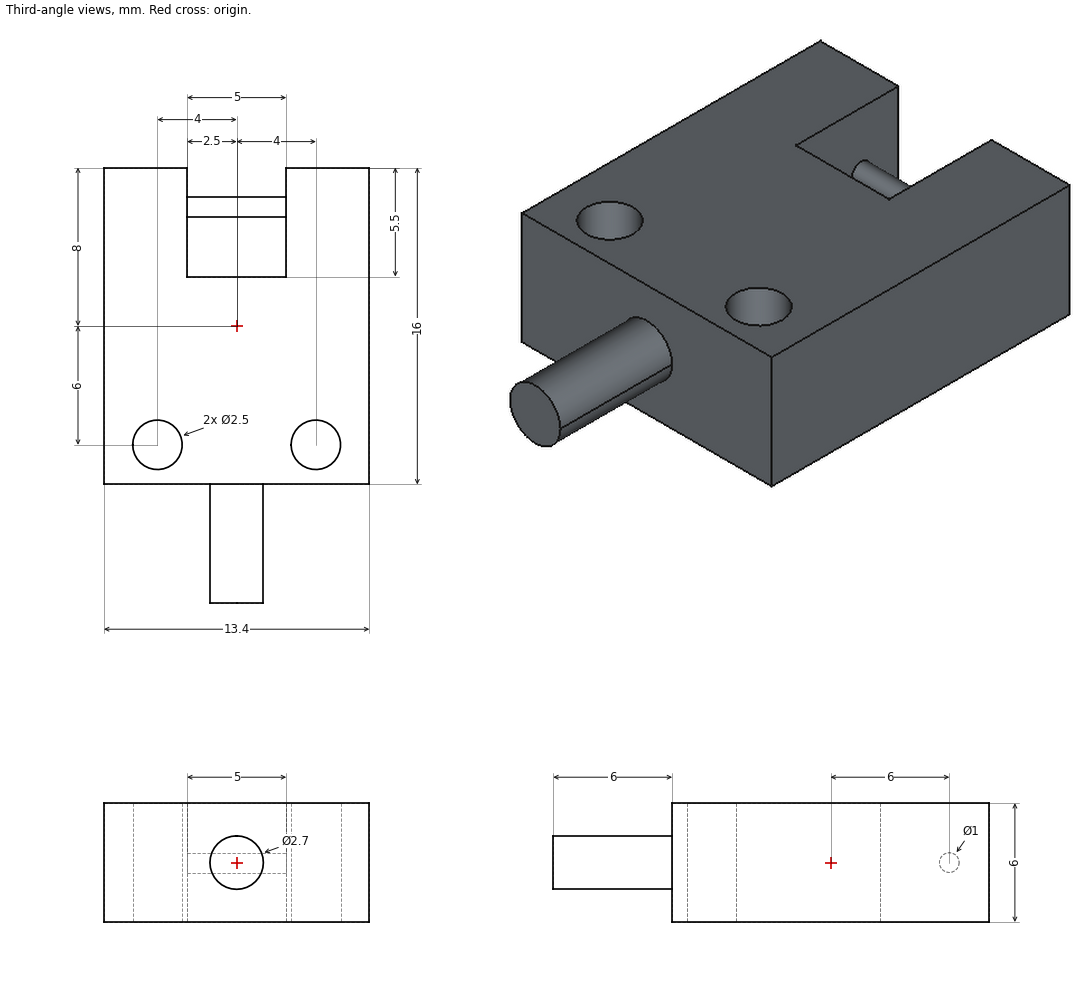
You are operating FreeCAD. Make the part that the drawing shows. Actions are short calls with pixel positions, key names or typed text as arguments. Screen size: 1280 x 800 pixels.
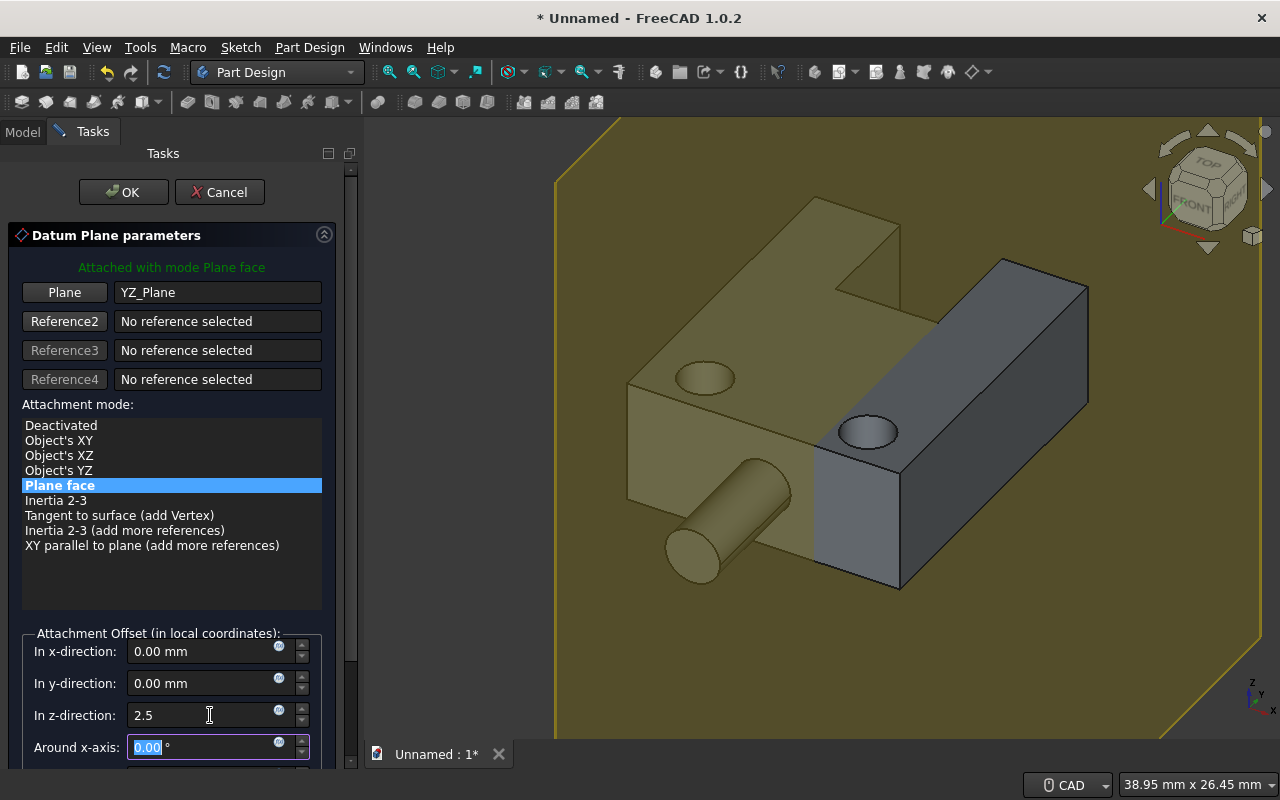
click(124, 192)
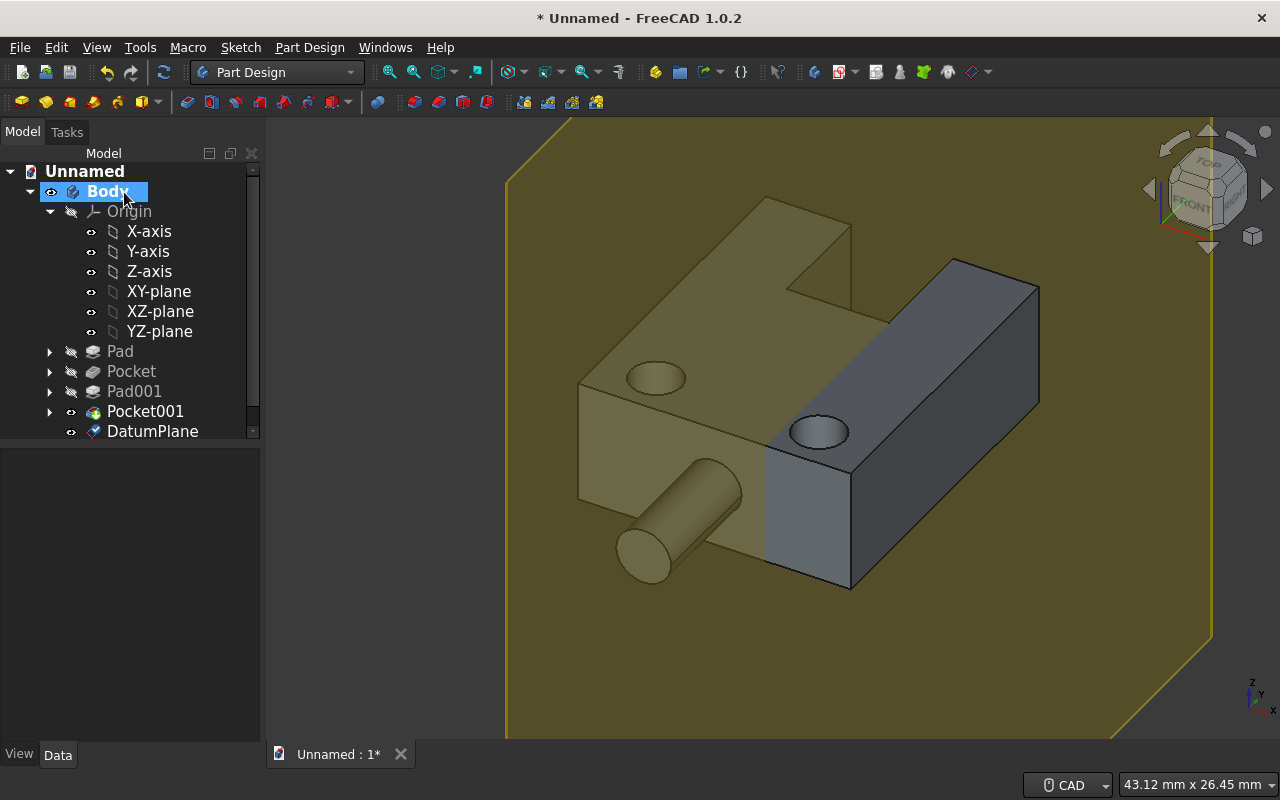
click(116, 432)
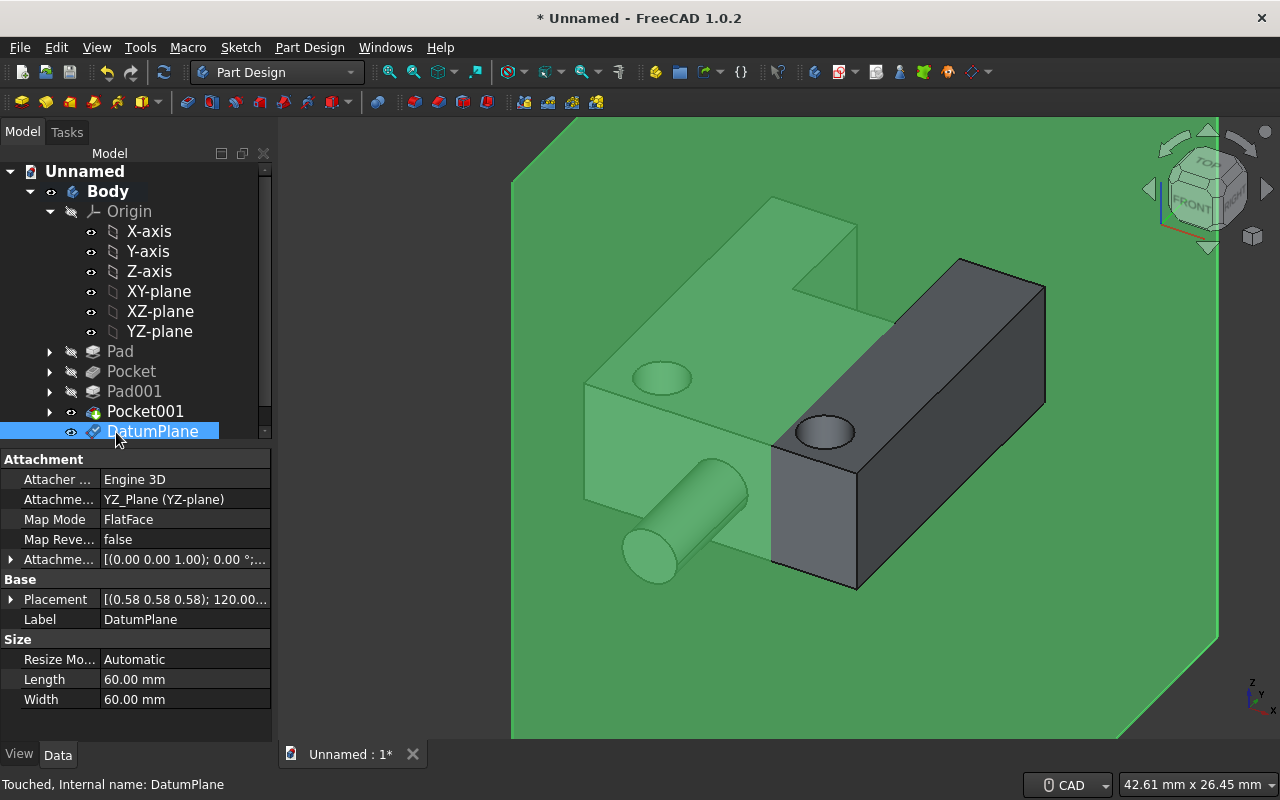
click(840, 72)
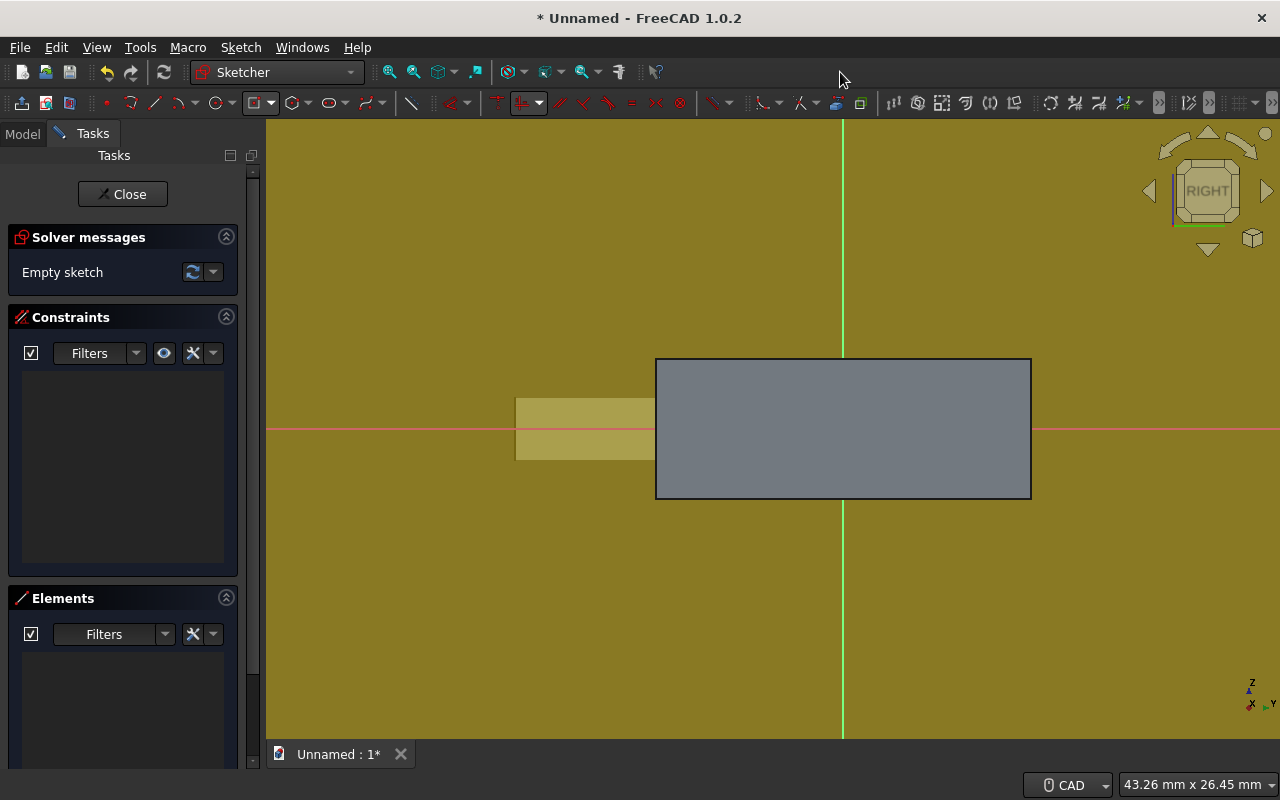
key(q)
key(s)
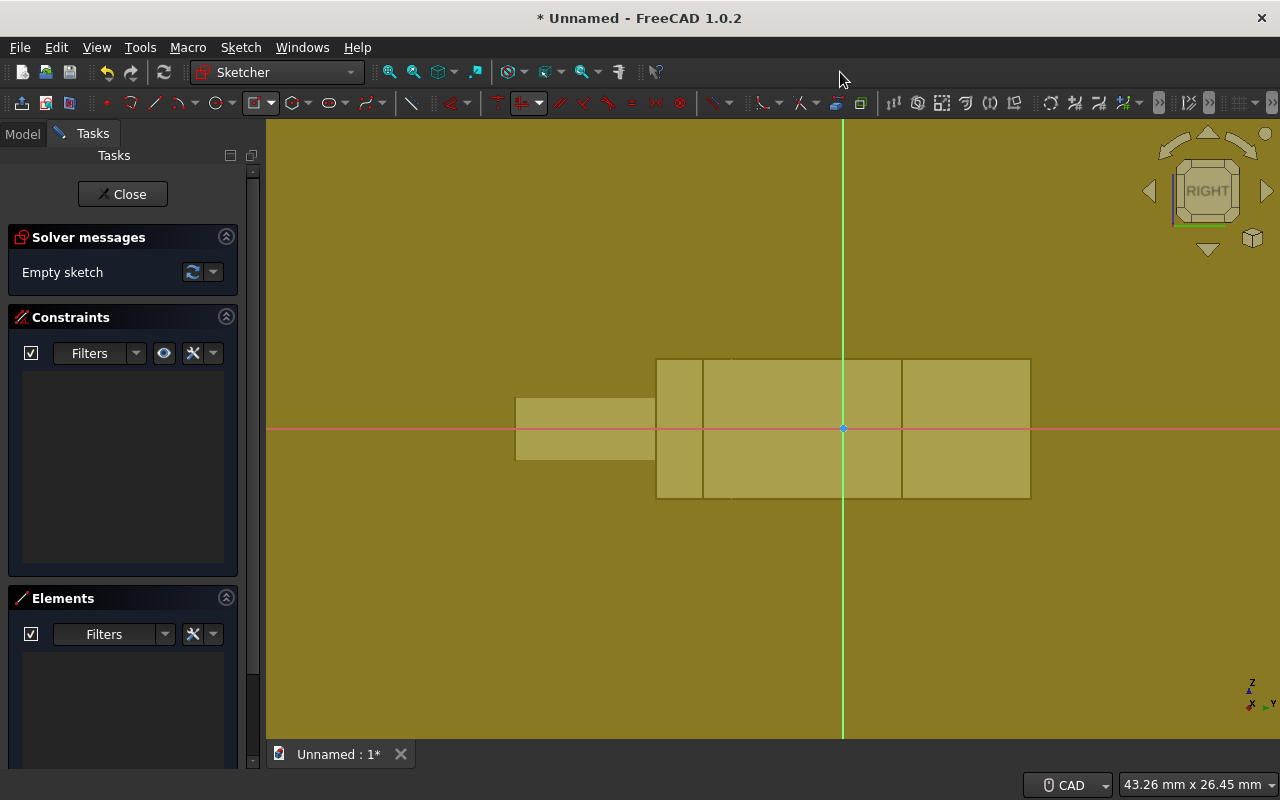
scroll(1002, 429, up, 14)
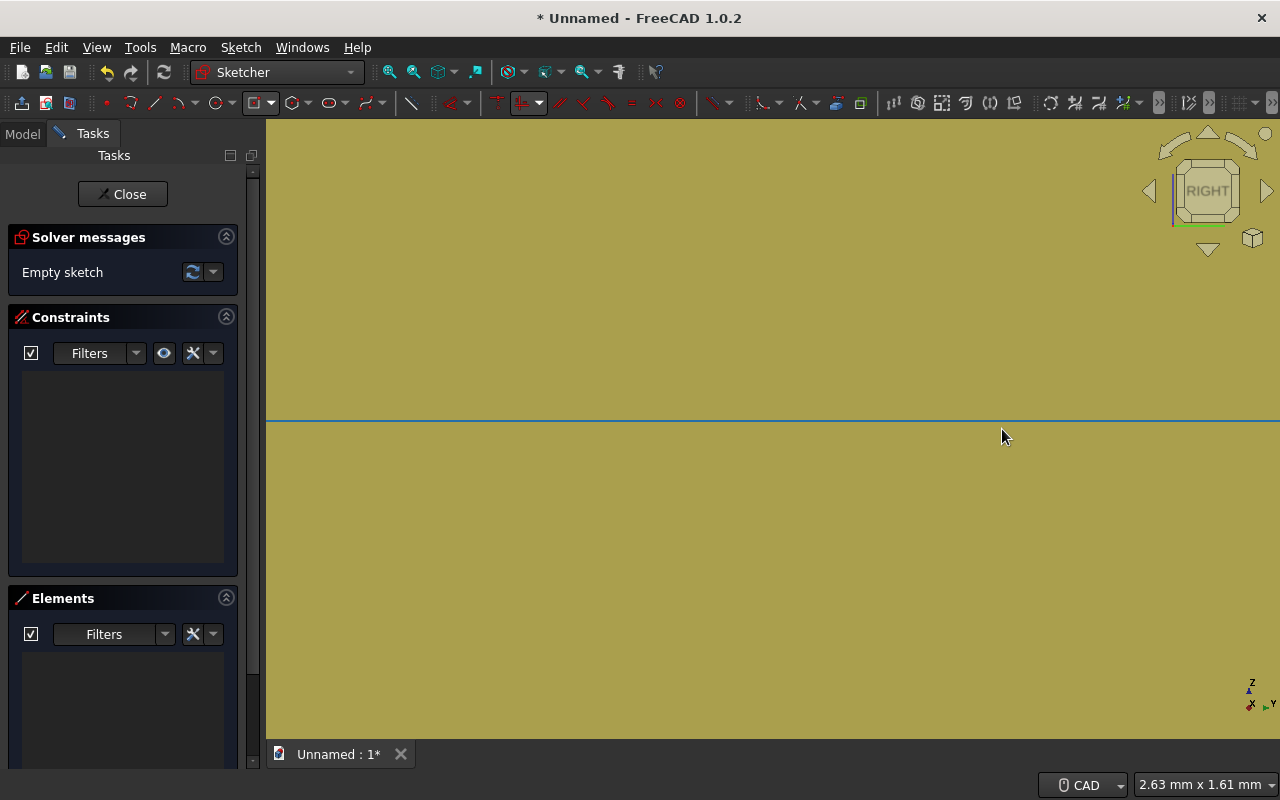
click(216, 104)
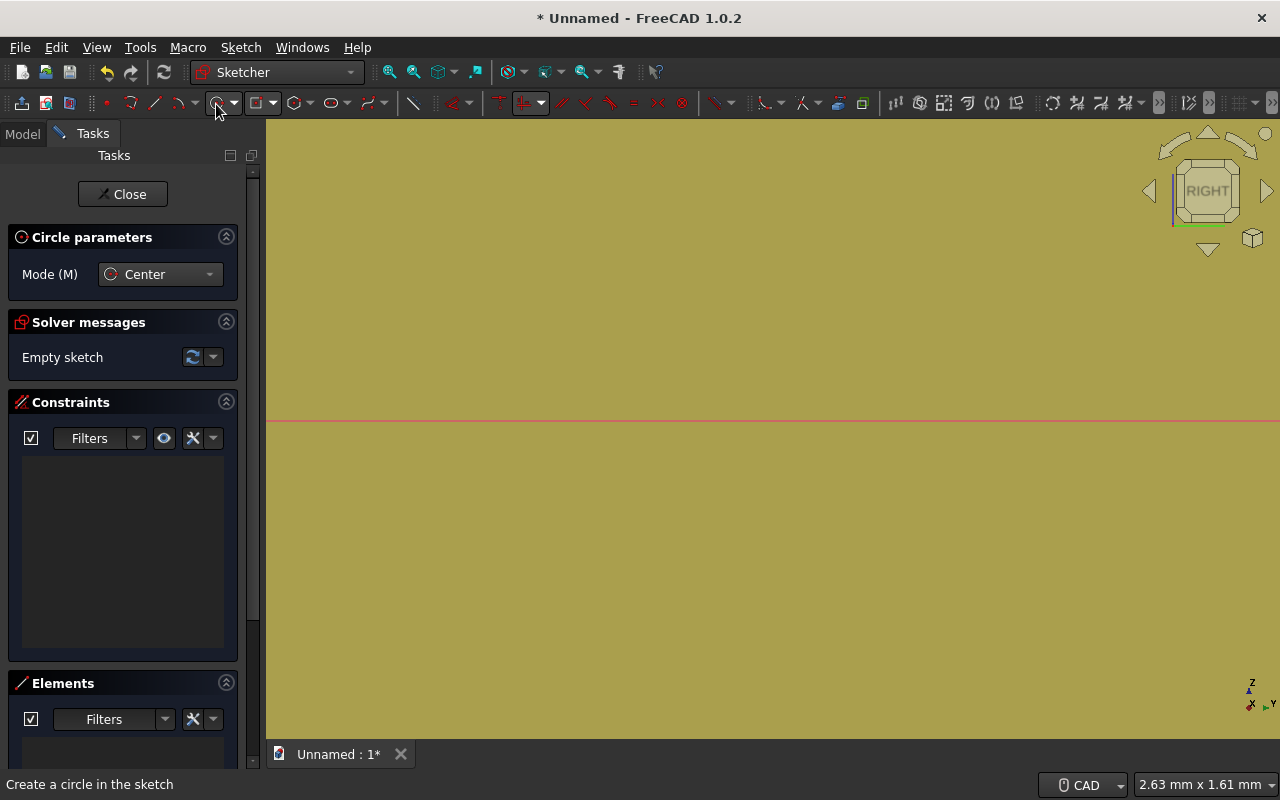
click(694, 421)
move(831, 285)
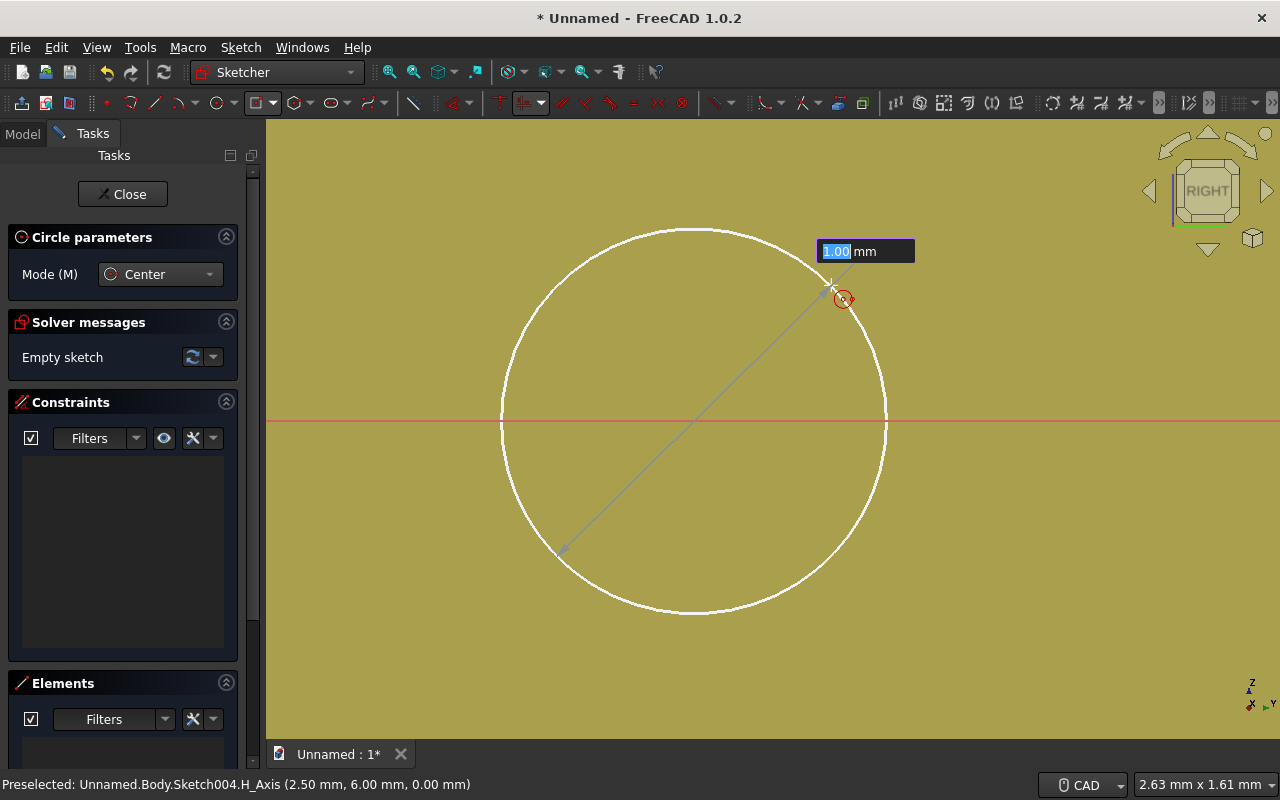
text(1)
key(Return)
key(Escape)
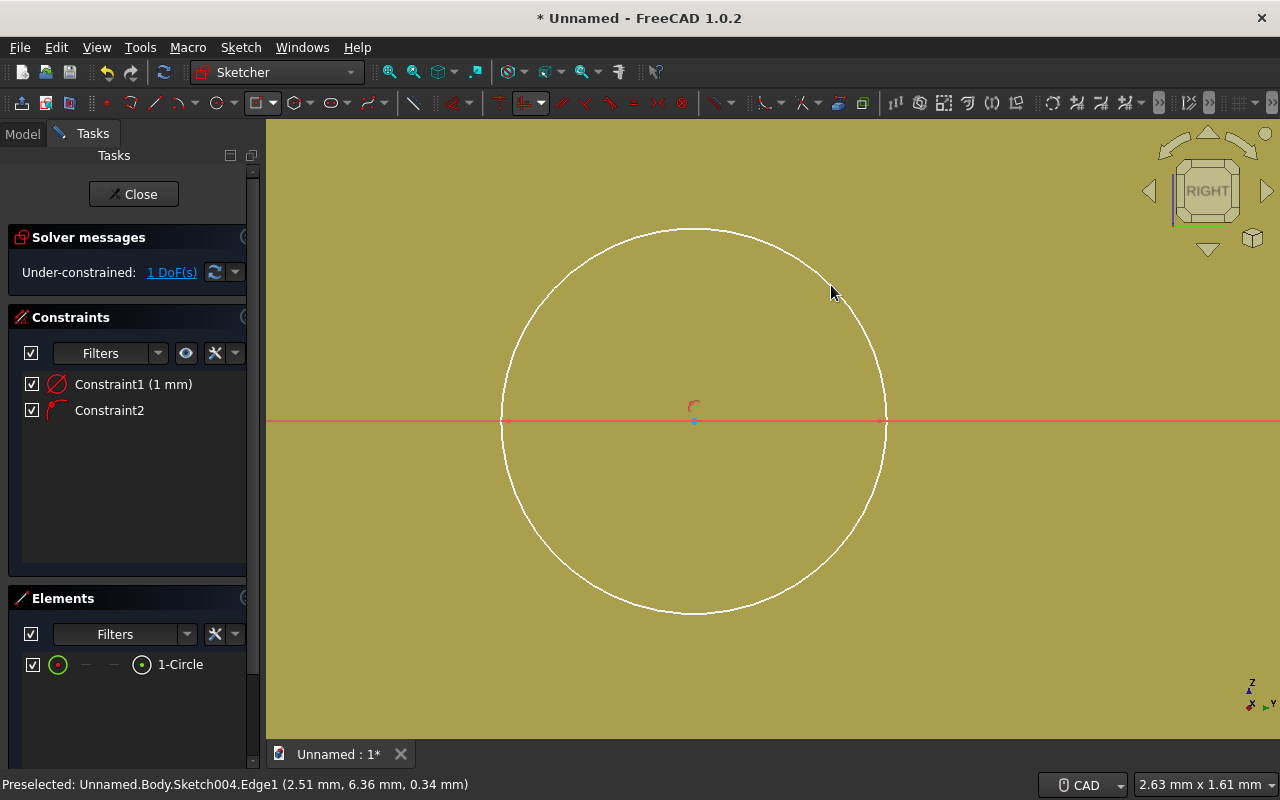
key(d)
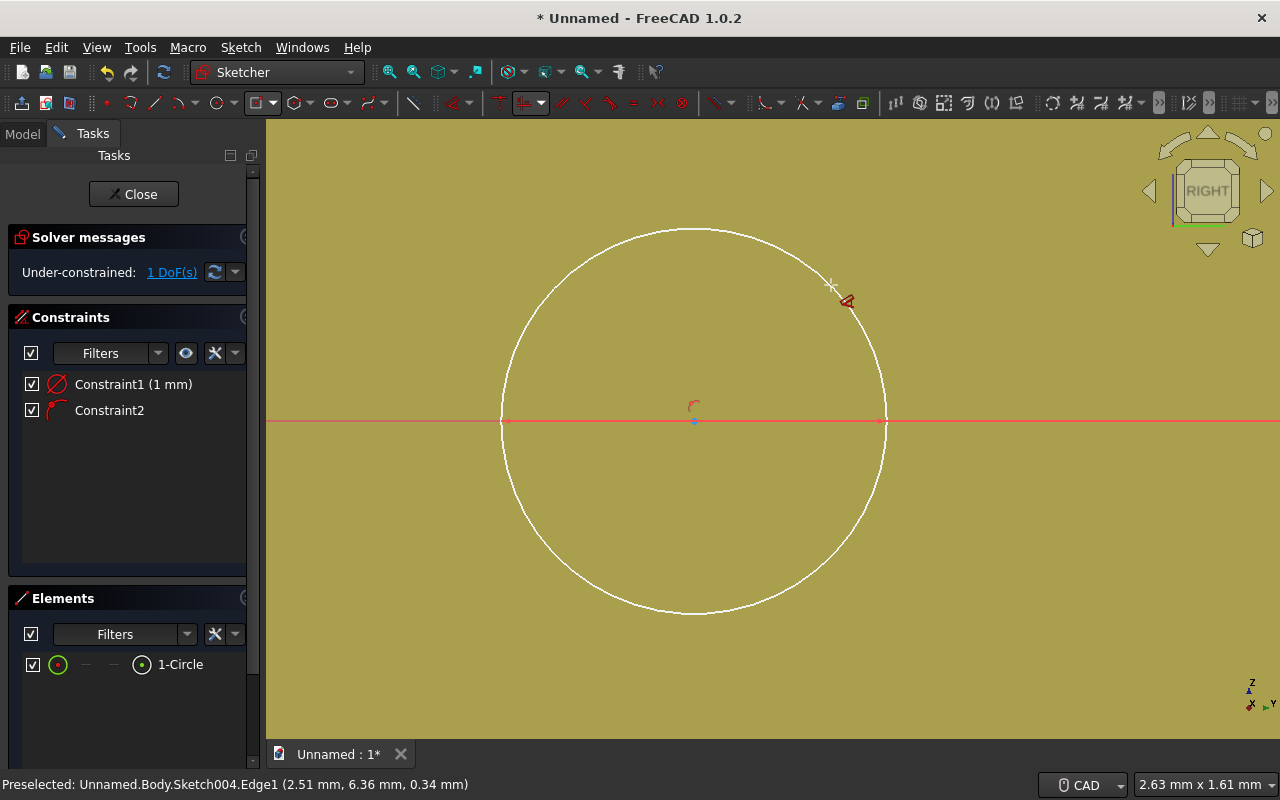
click(694, 421)
click(402, 455)